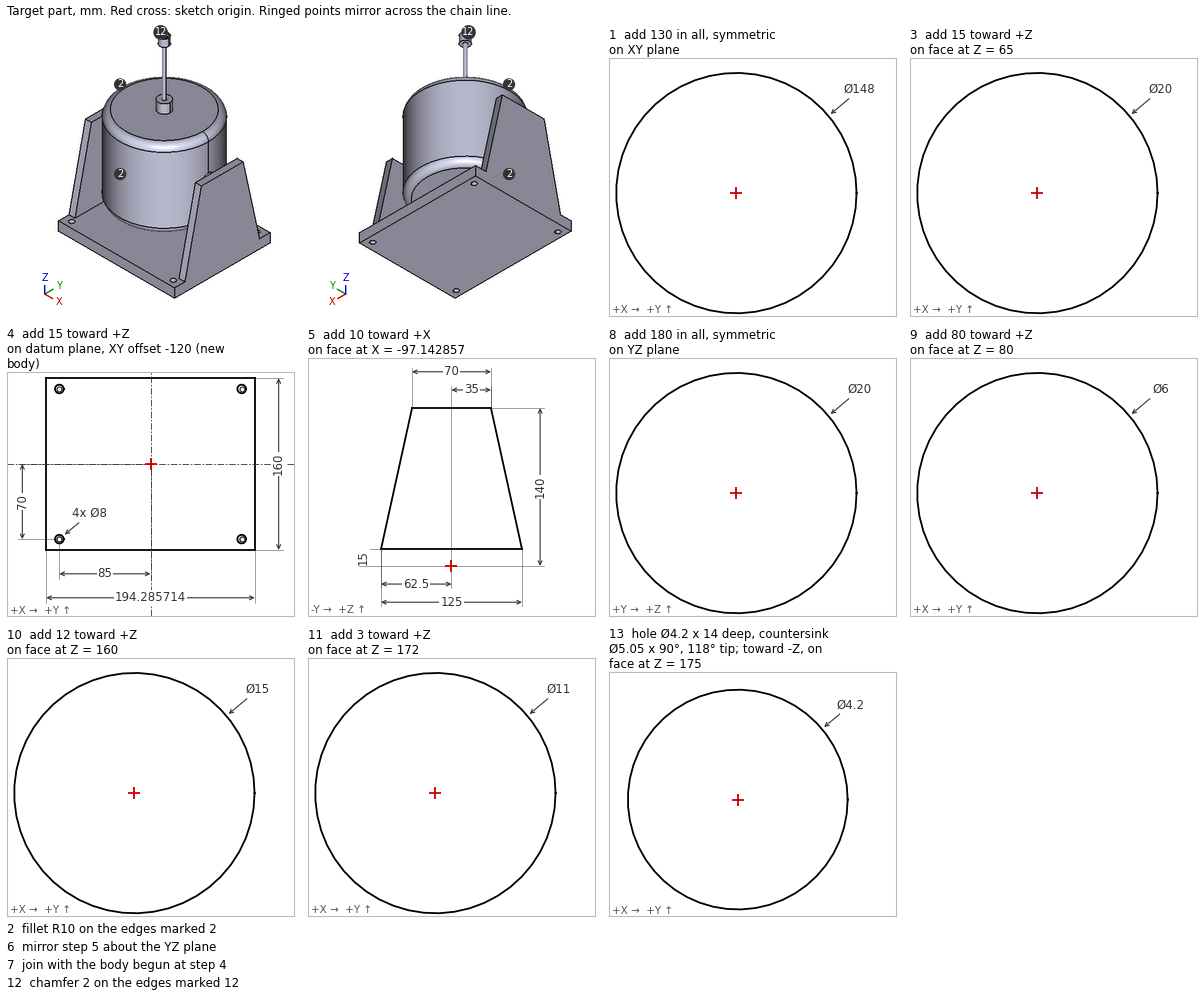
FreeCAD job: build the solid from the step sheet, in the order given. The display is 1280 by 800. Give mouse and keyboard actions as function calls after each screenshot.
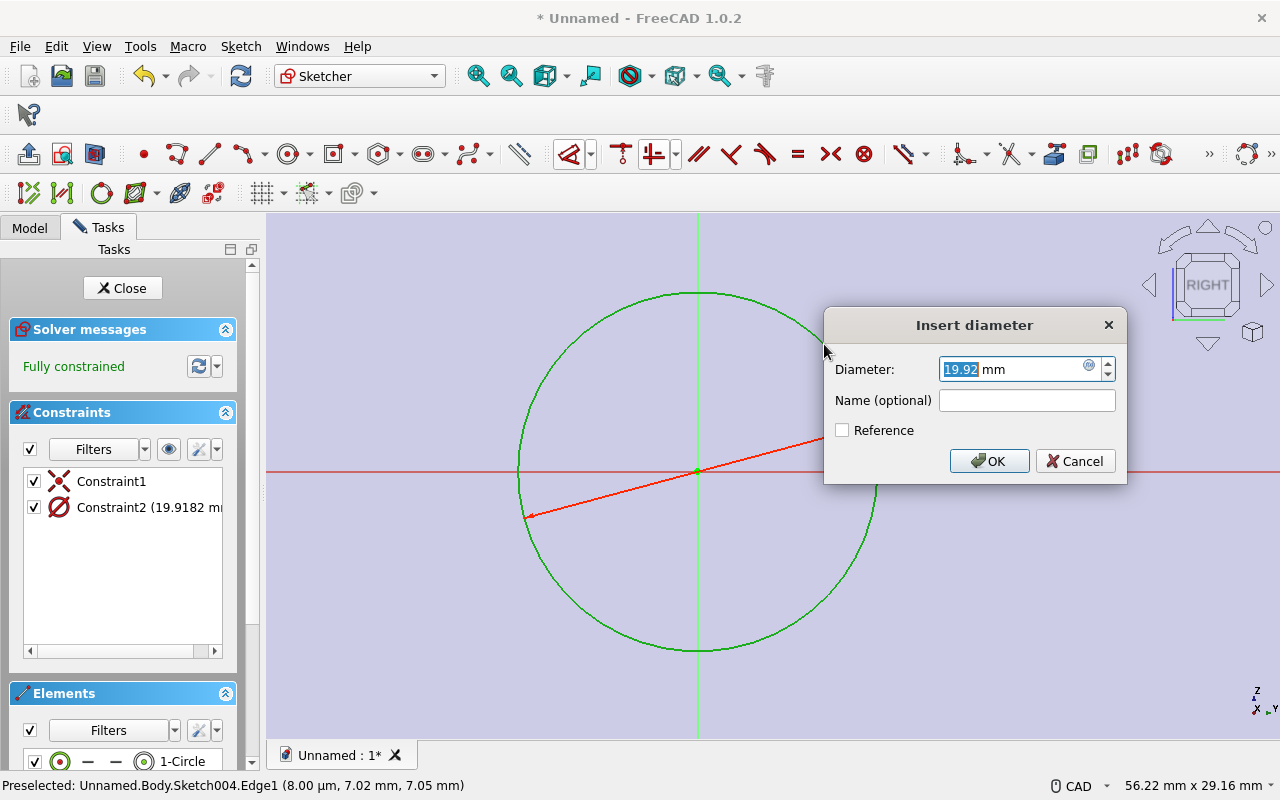
text(20)
key(Return)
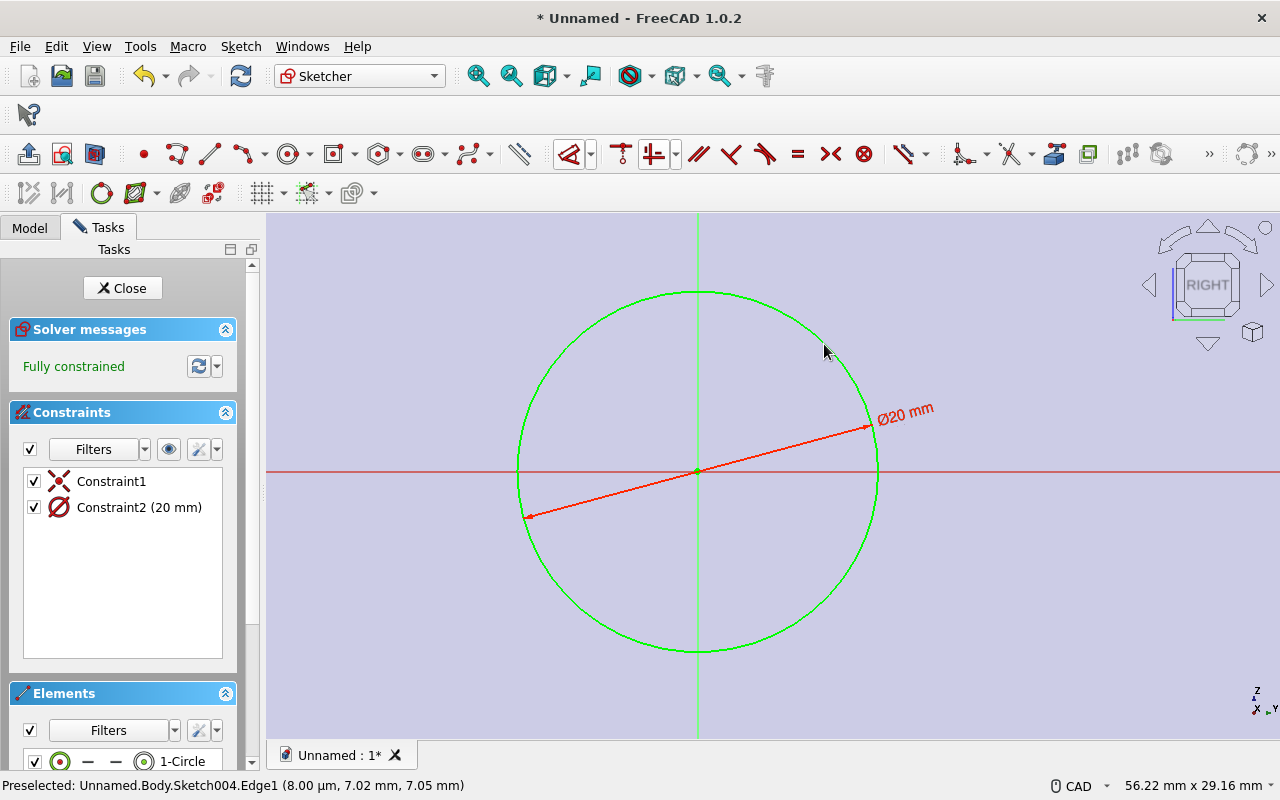
click(123, 288)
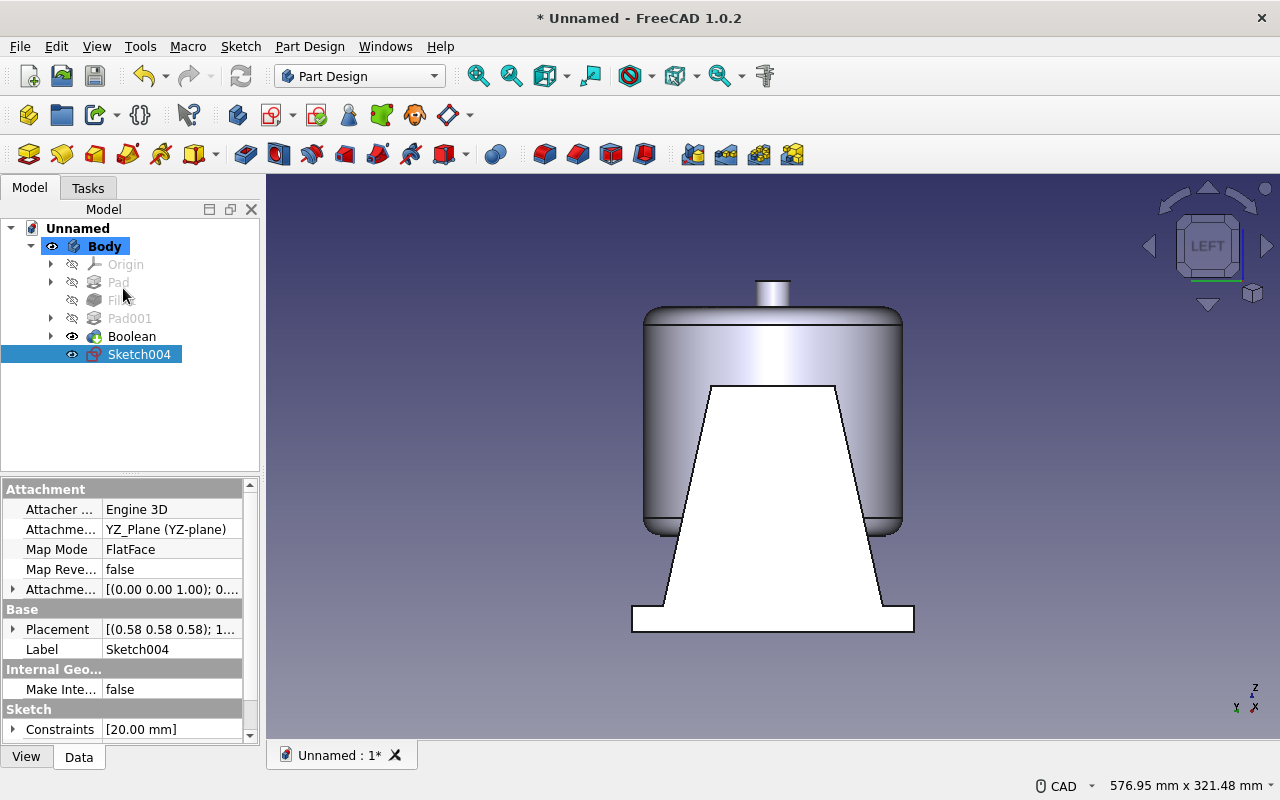
click(29, 154)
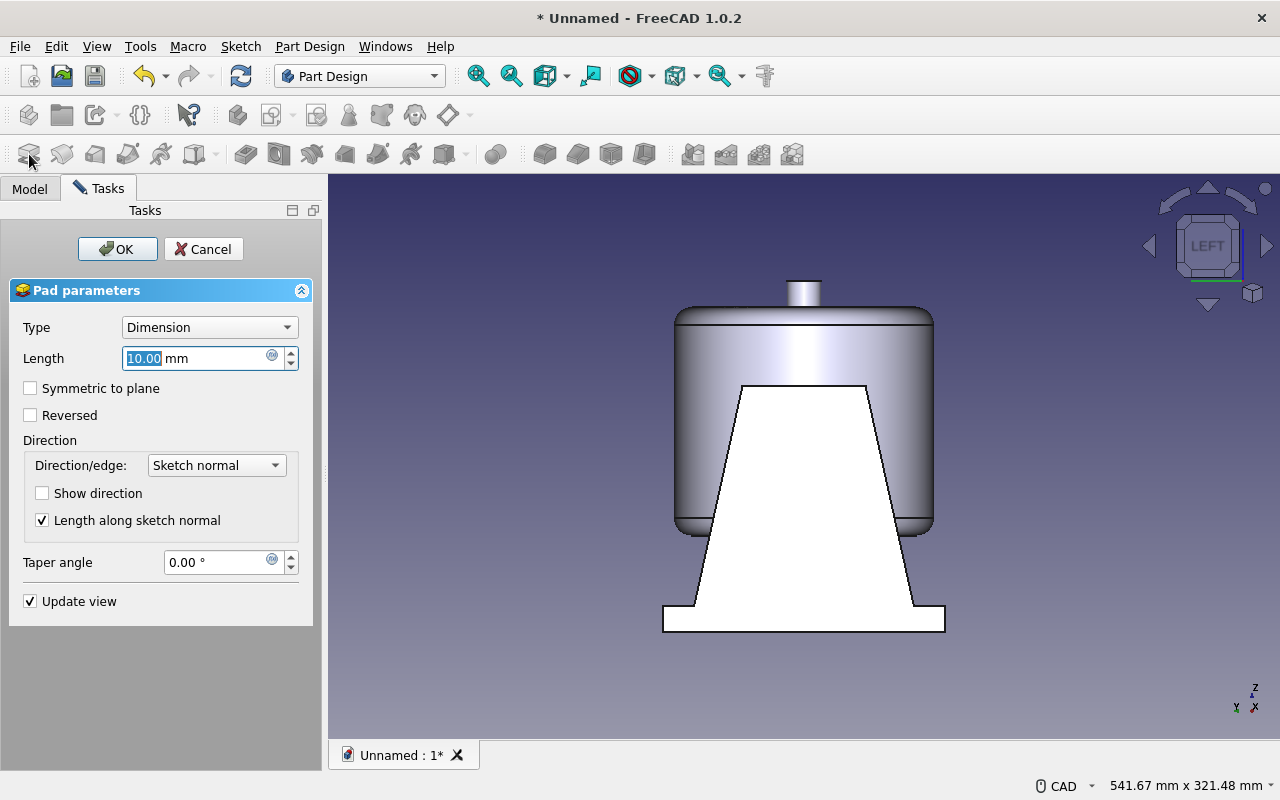
text(180)
key(Tab)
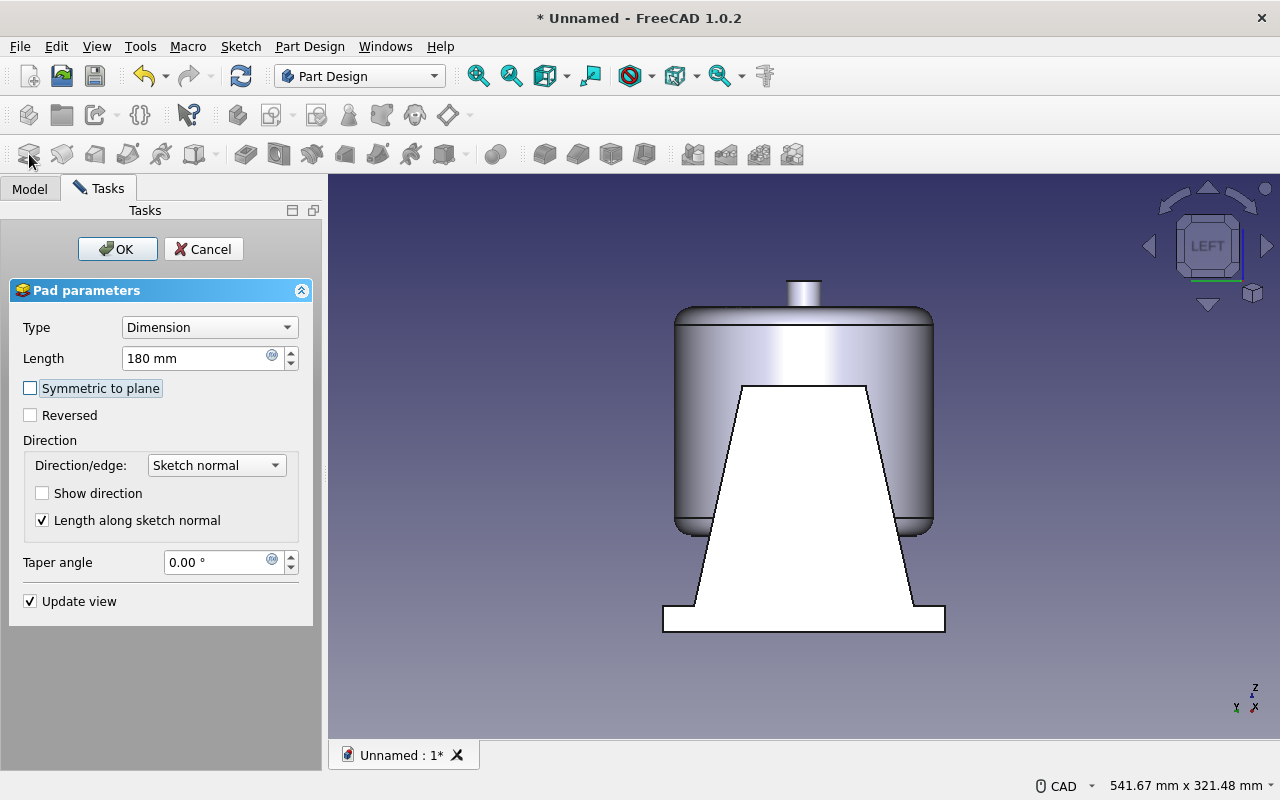
click(31, 388)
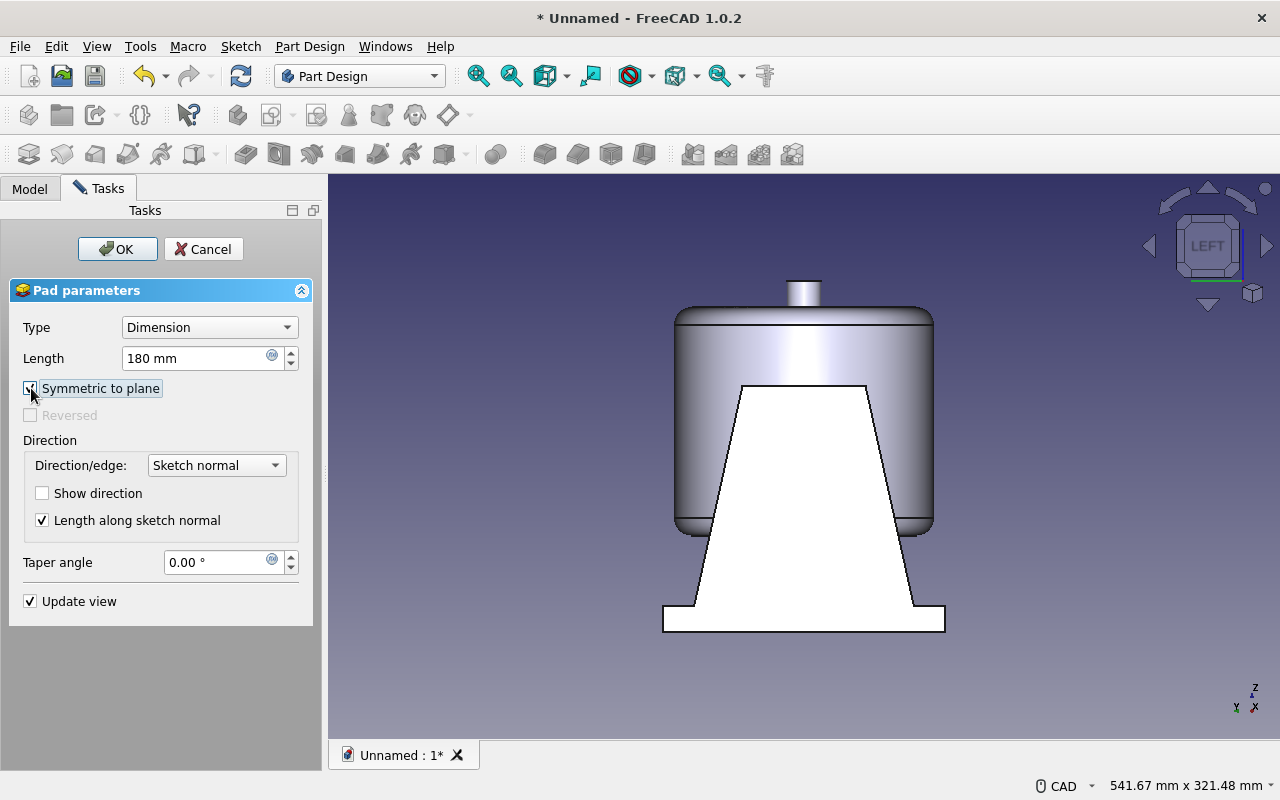
click(118, 249)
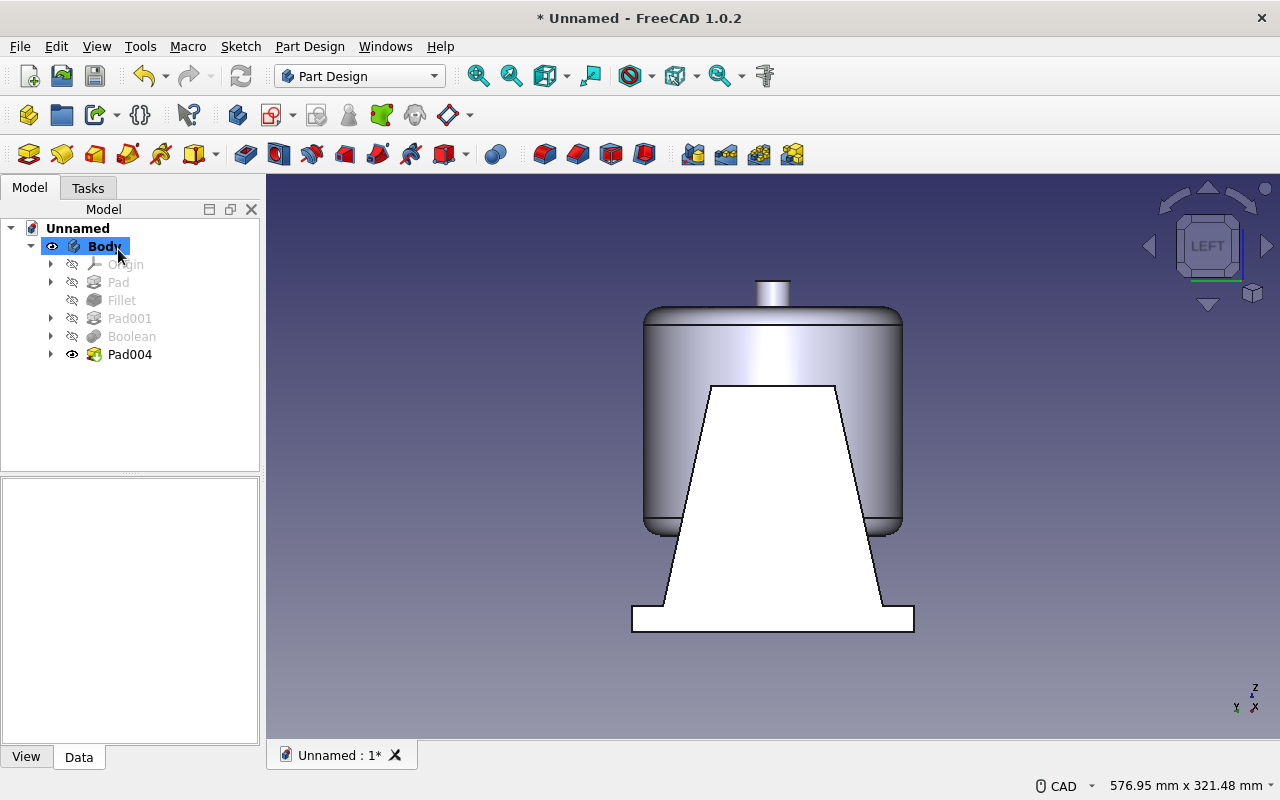
key(0)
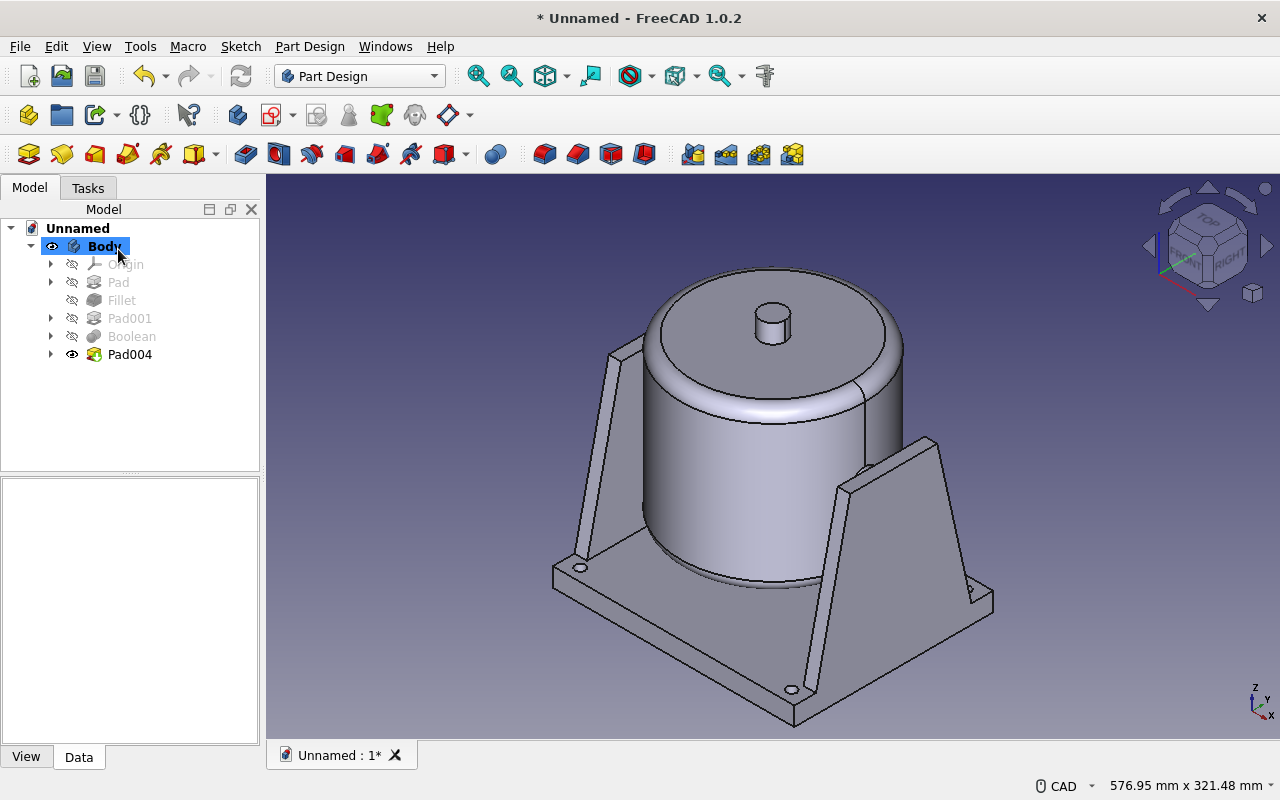
click(773, 312)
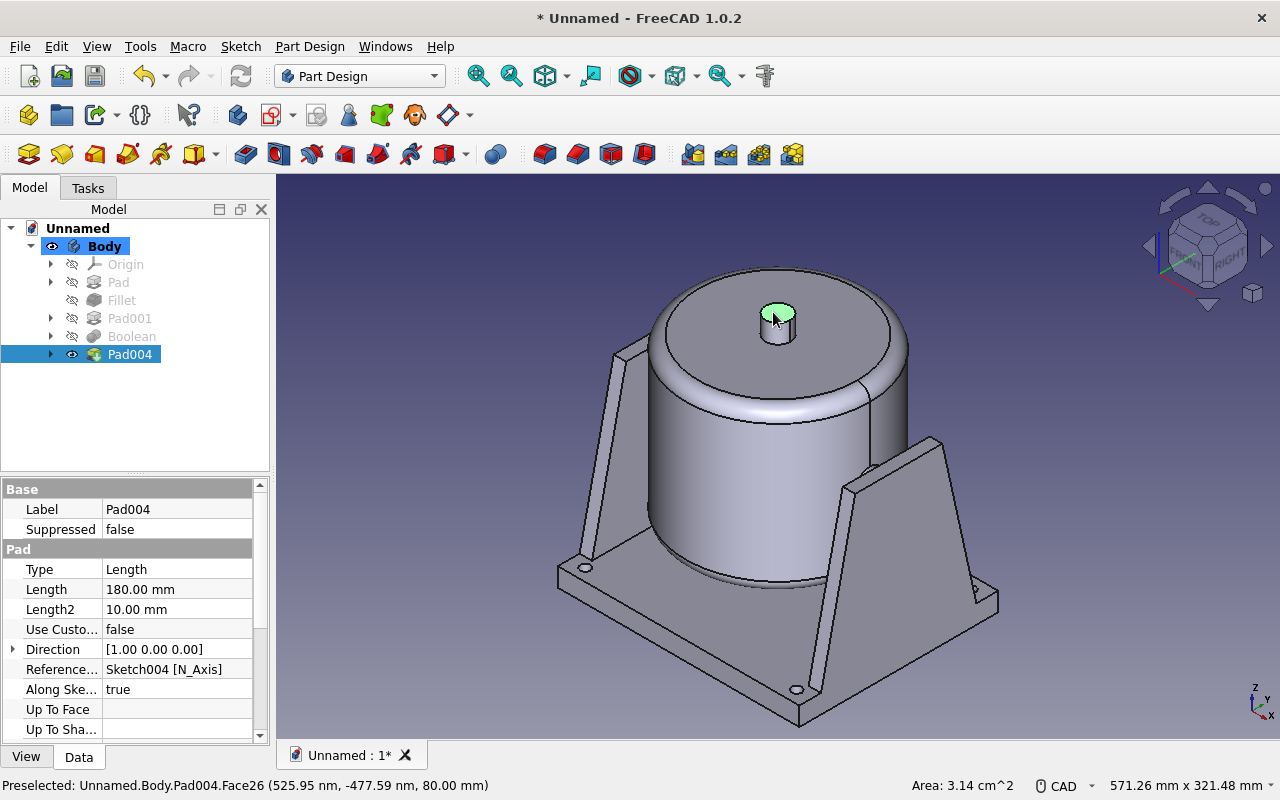
click(270, 116)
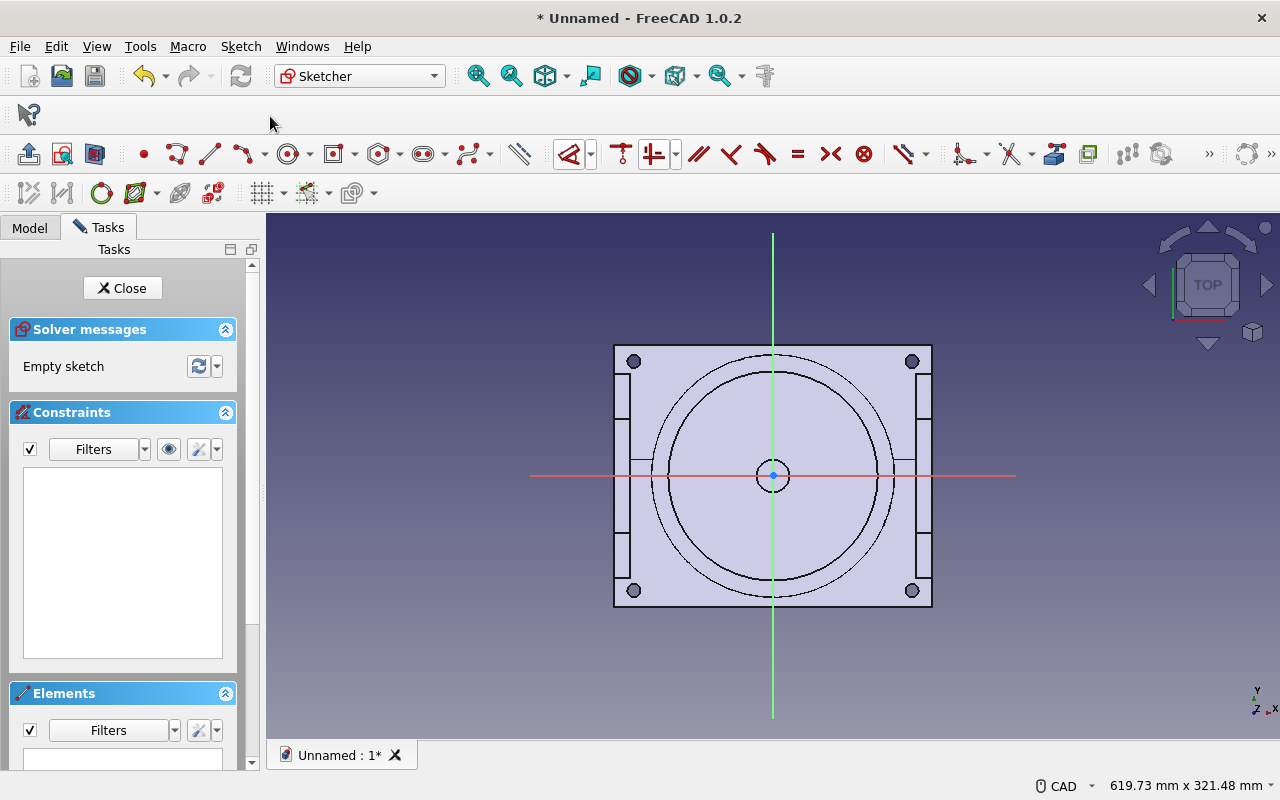
scroll(777, 476, up, 15)